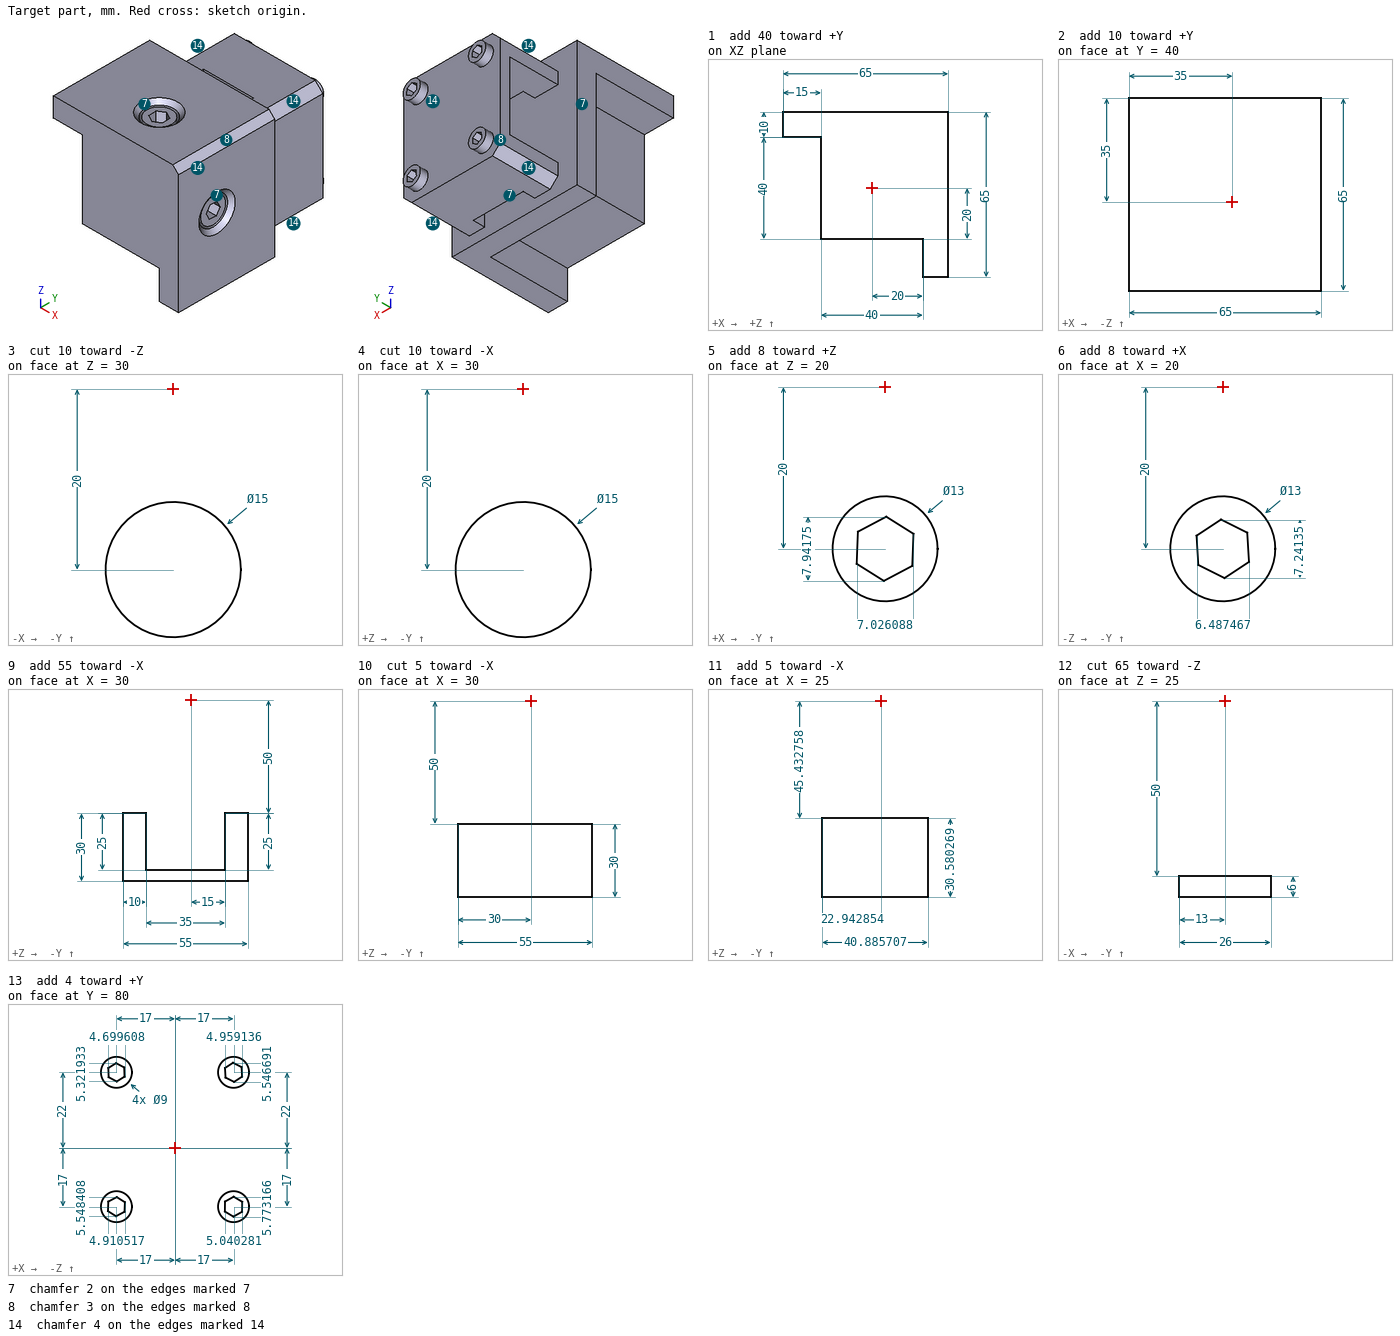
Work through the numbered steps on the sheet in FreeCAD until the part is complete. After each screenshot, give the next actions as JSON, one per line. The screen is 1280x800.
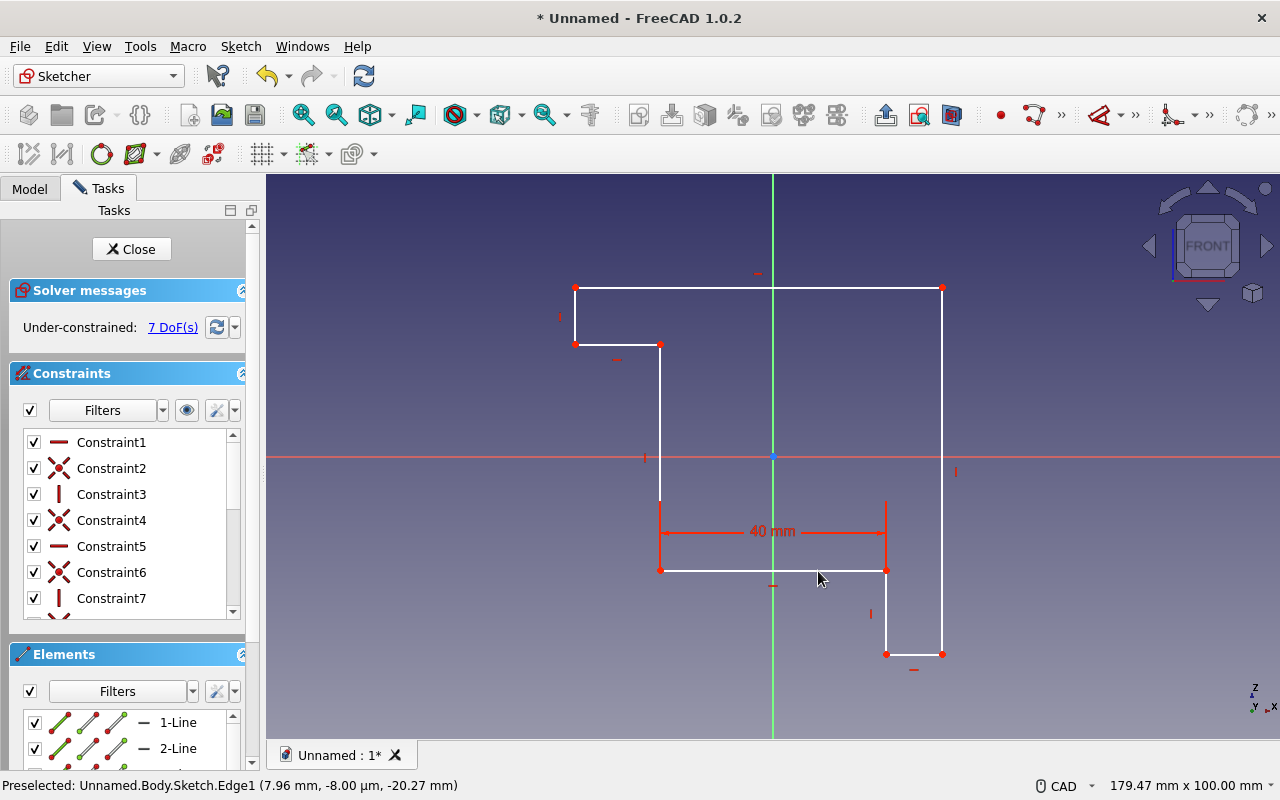
{"action": "left_click", "coordinate": [660, 503]}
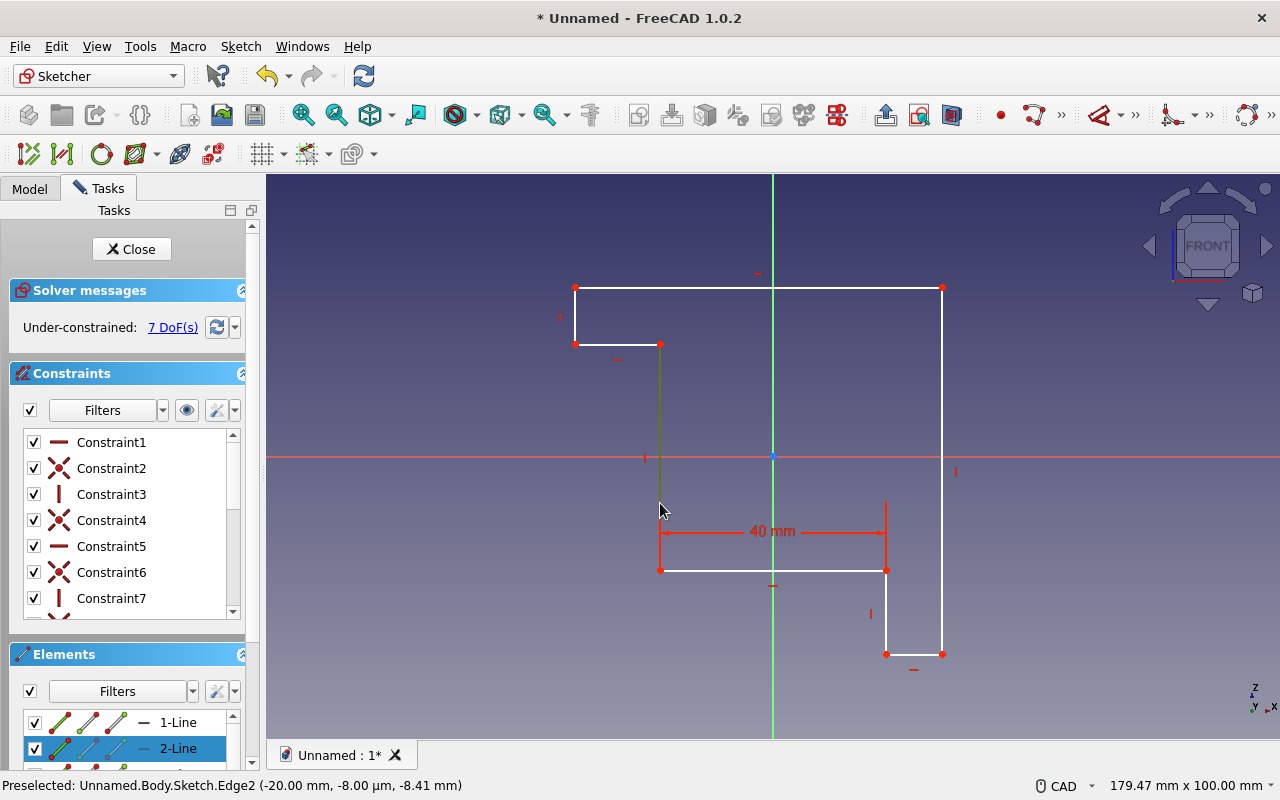
{"action": "left_click", "coordinate": [1120, 116]}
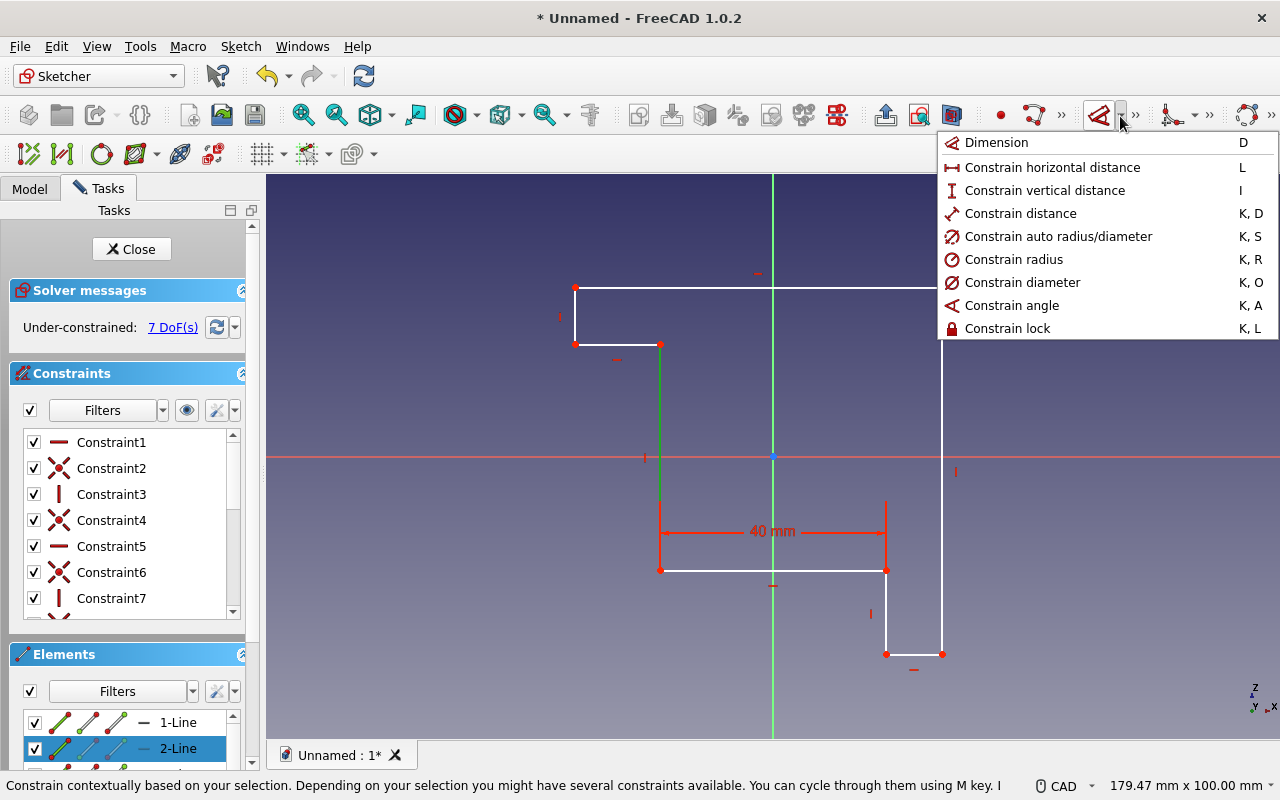
{"action": "left_click", "coordinate": [1108, 190]}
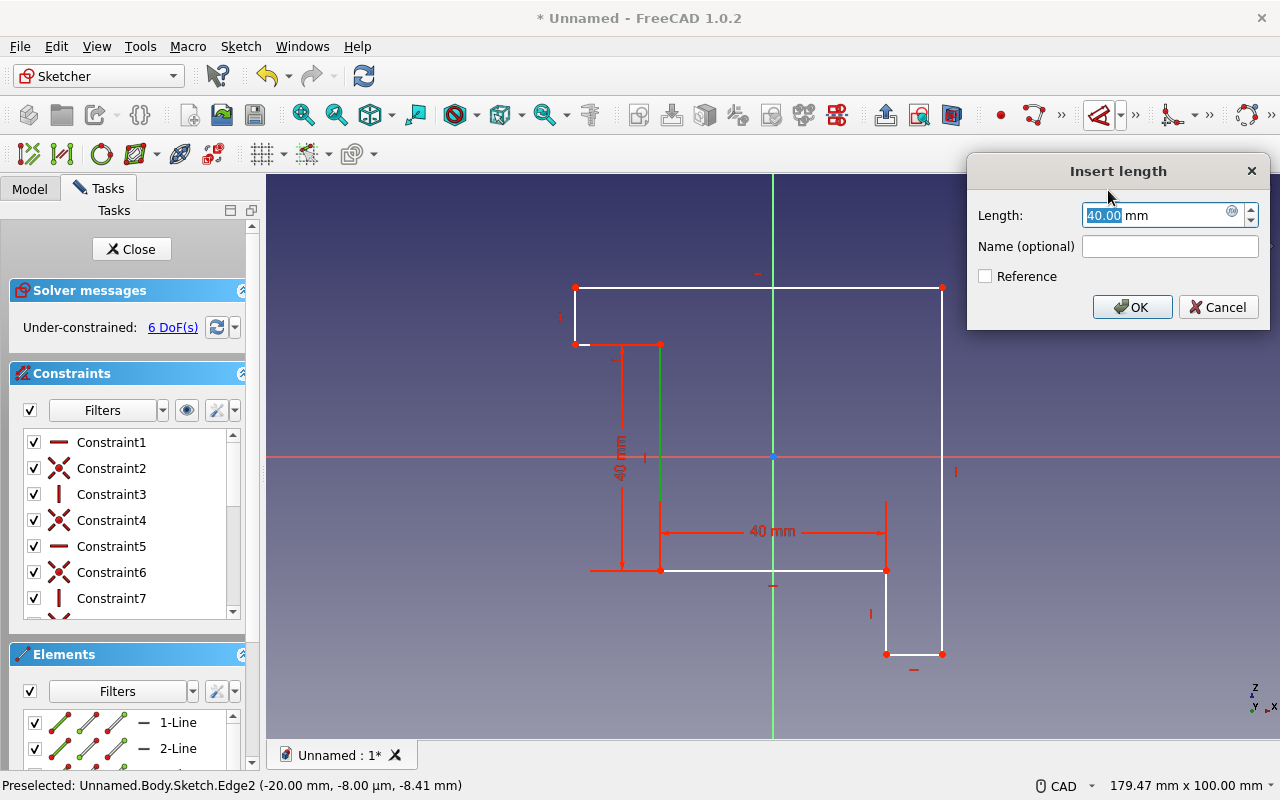
{"action": "type", "text": "40"}
{"action": "key", "text": "Return"}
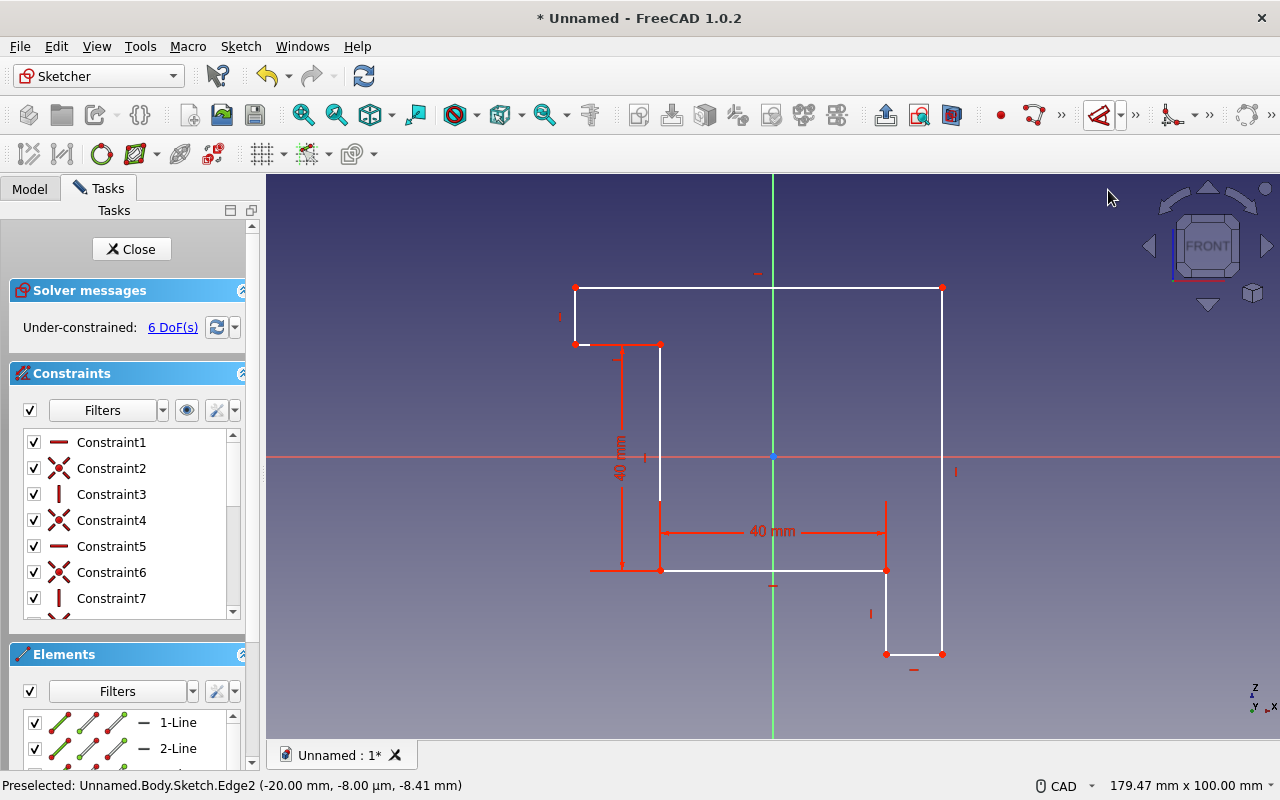
{"action": "left_click", "coordinate": [634, 345]}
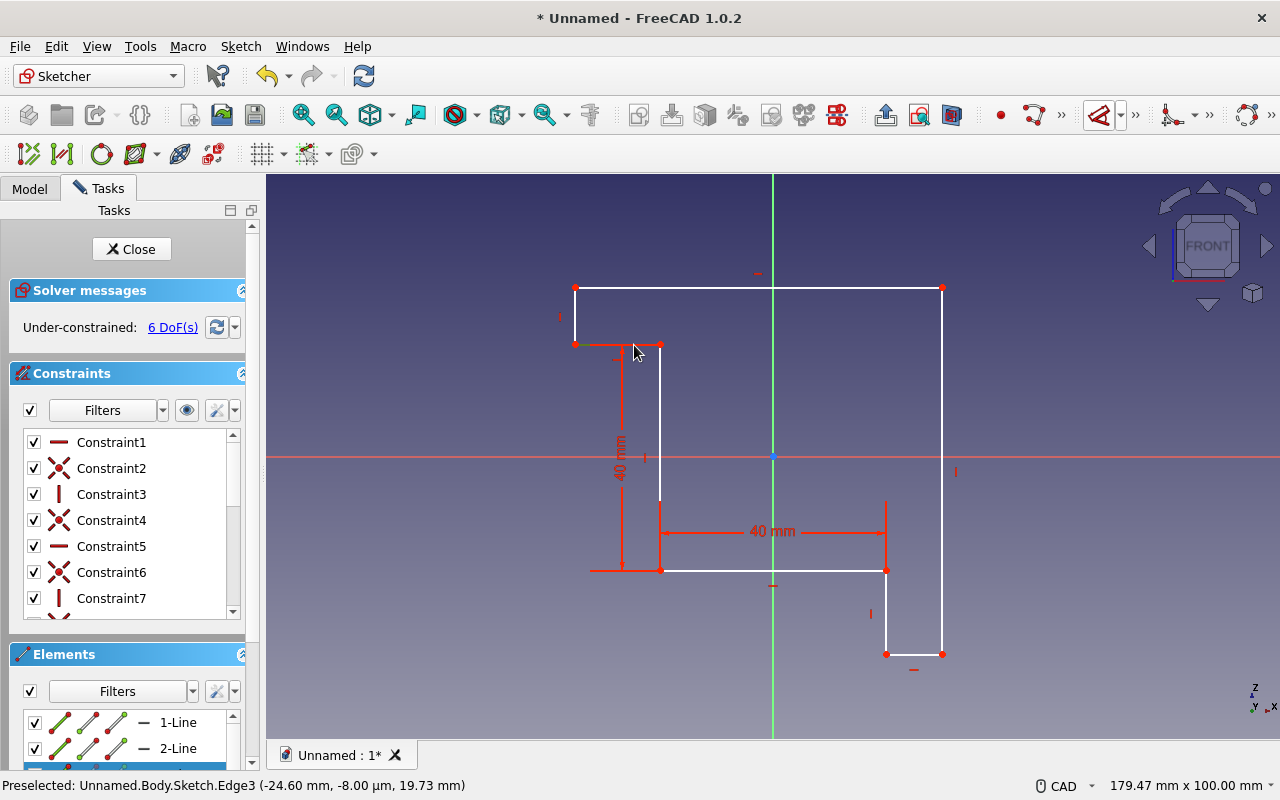
{"action": "key", "text": "l"}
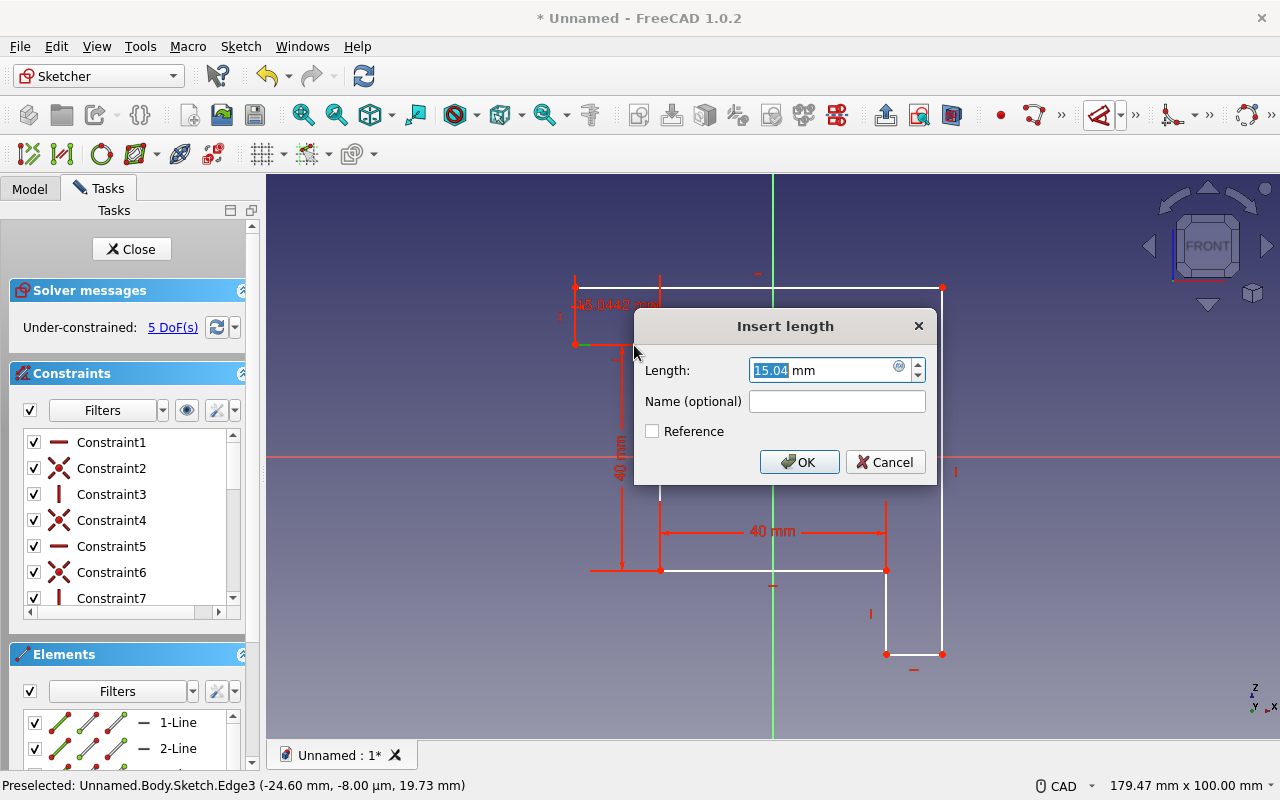
{"action": "type", "text": "15"}
{"action": "key", "text": "Return"}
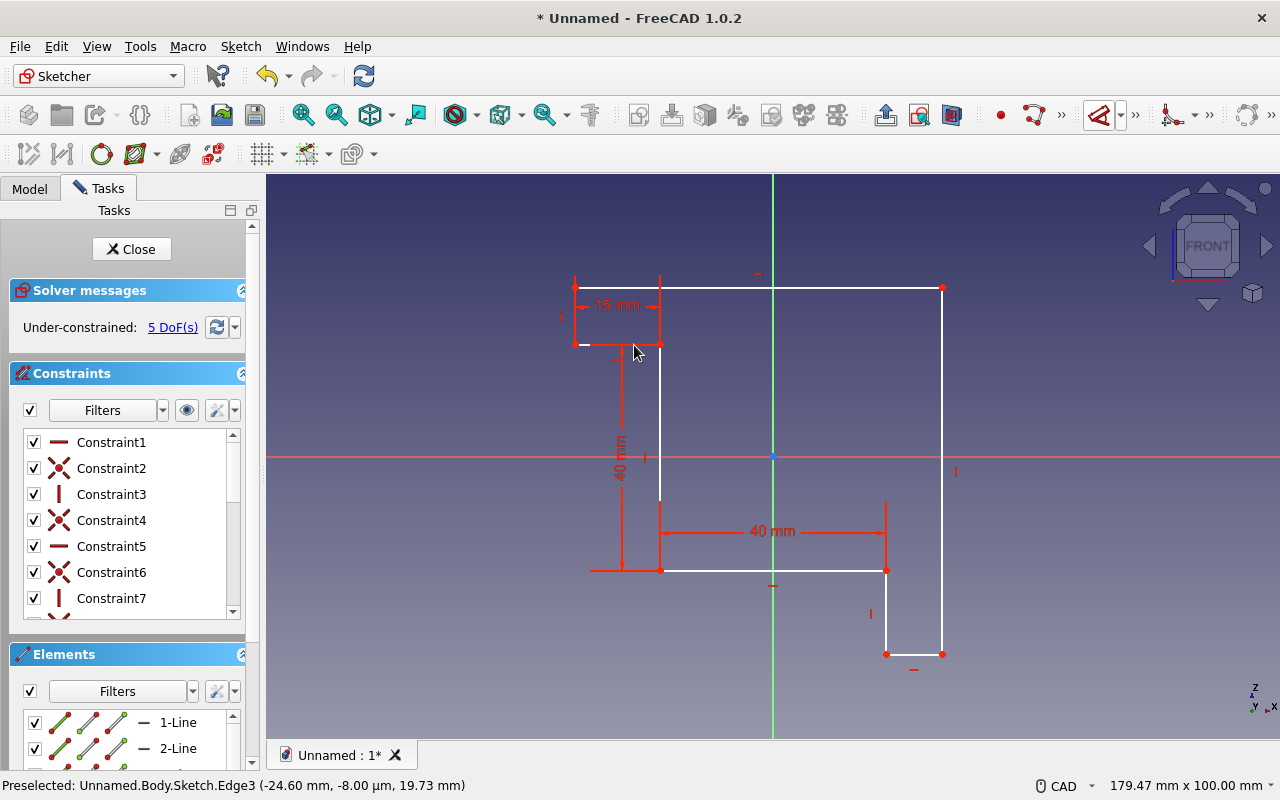
{"action": "left_click", "coordinate": [575, 328]}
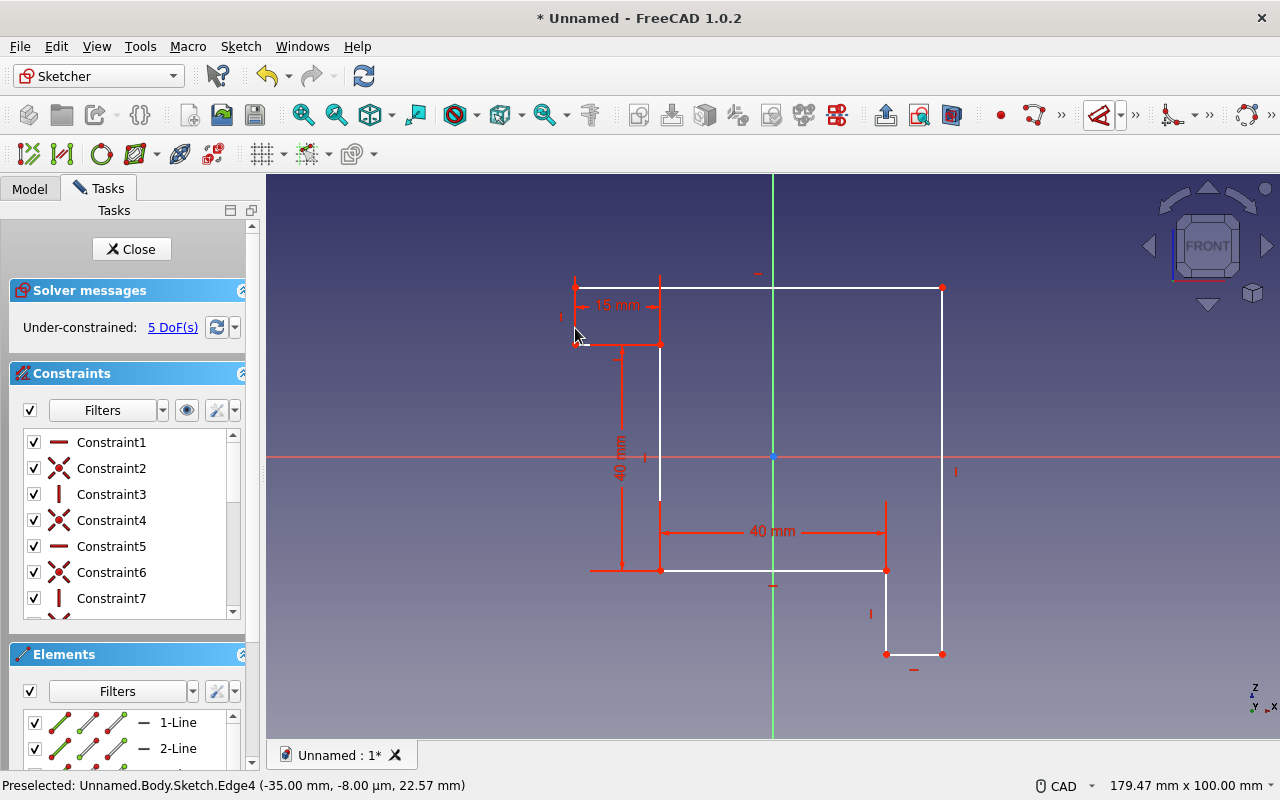
{"action": "left_click", "coordinate": [1120, 116]}